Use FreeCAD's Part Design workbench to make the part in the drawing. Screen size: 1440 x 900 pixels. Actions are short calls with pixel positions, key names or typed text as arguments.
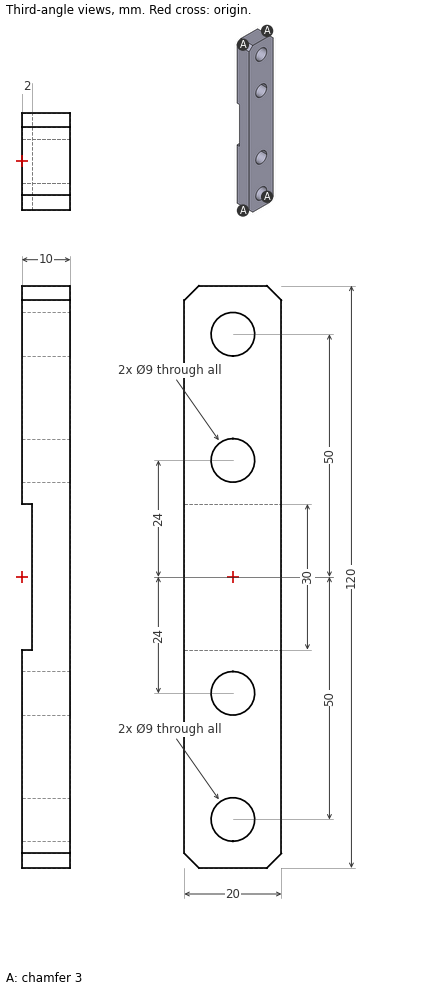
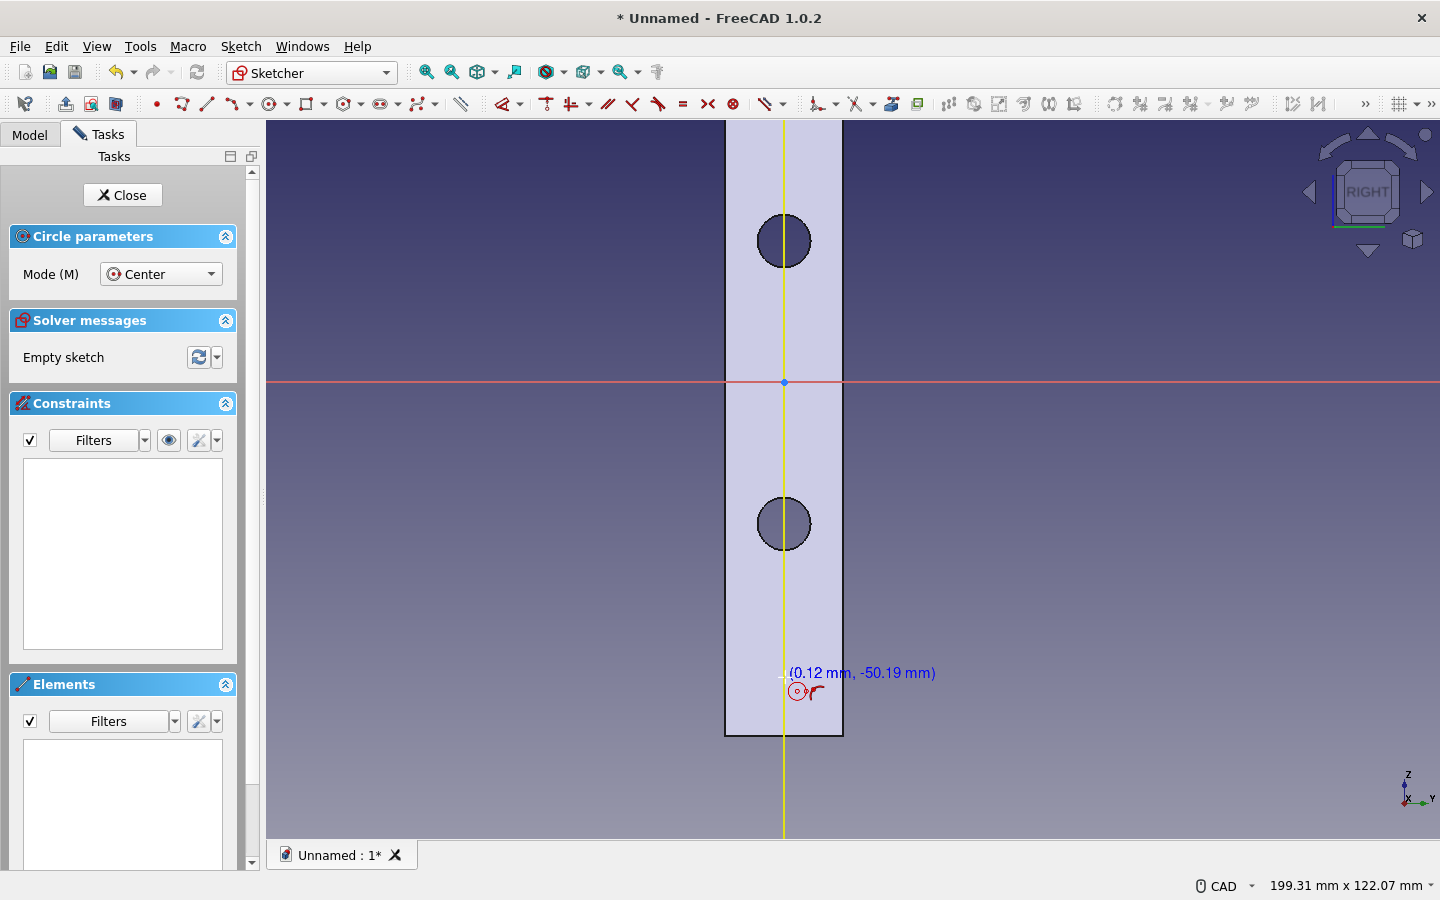
click(784, 677)
move(803, 658)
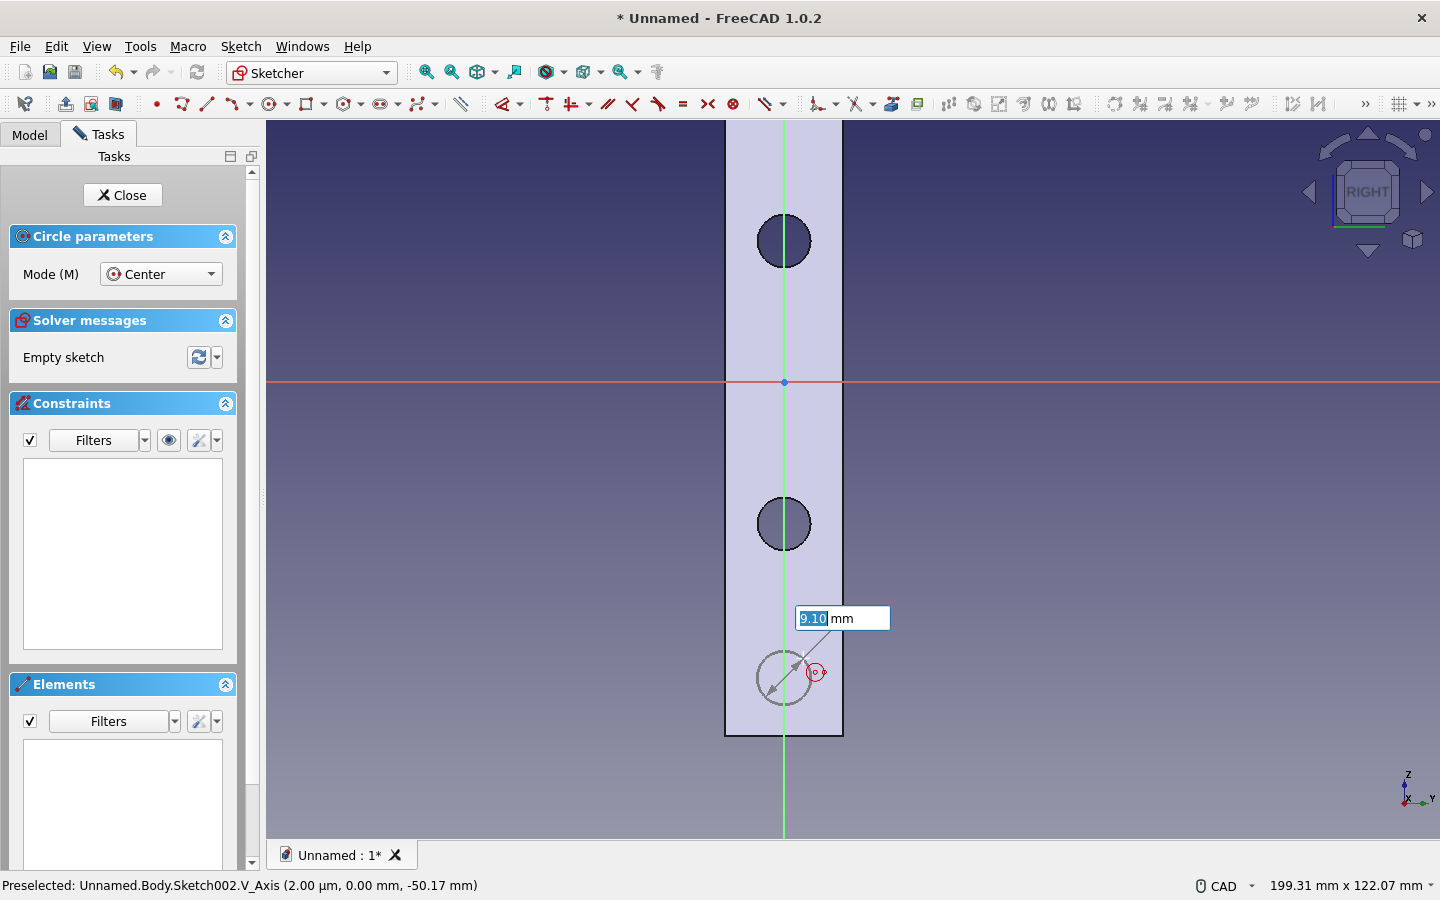
text(9)
key(Return)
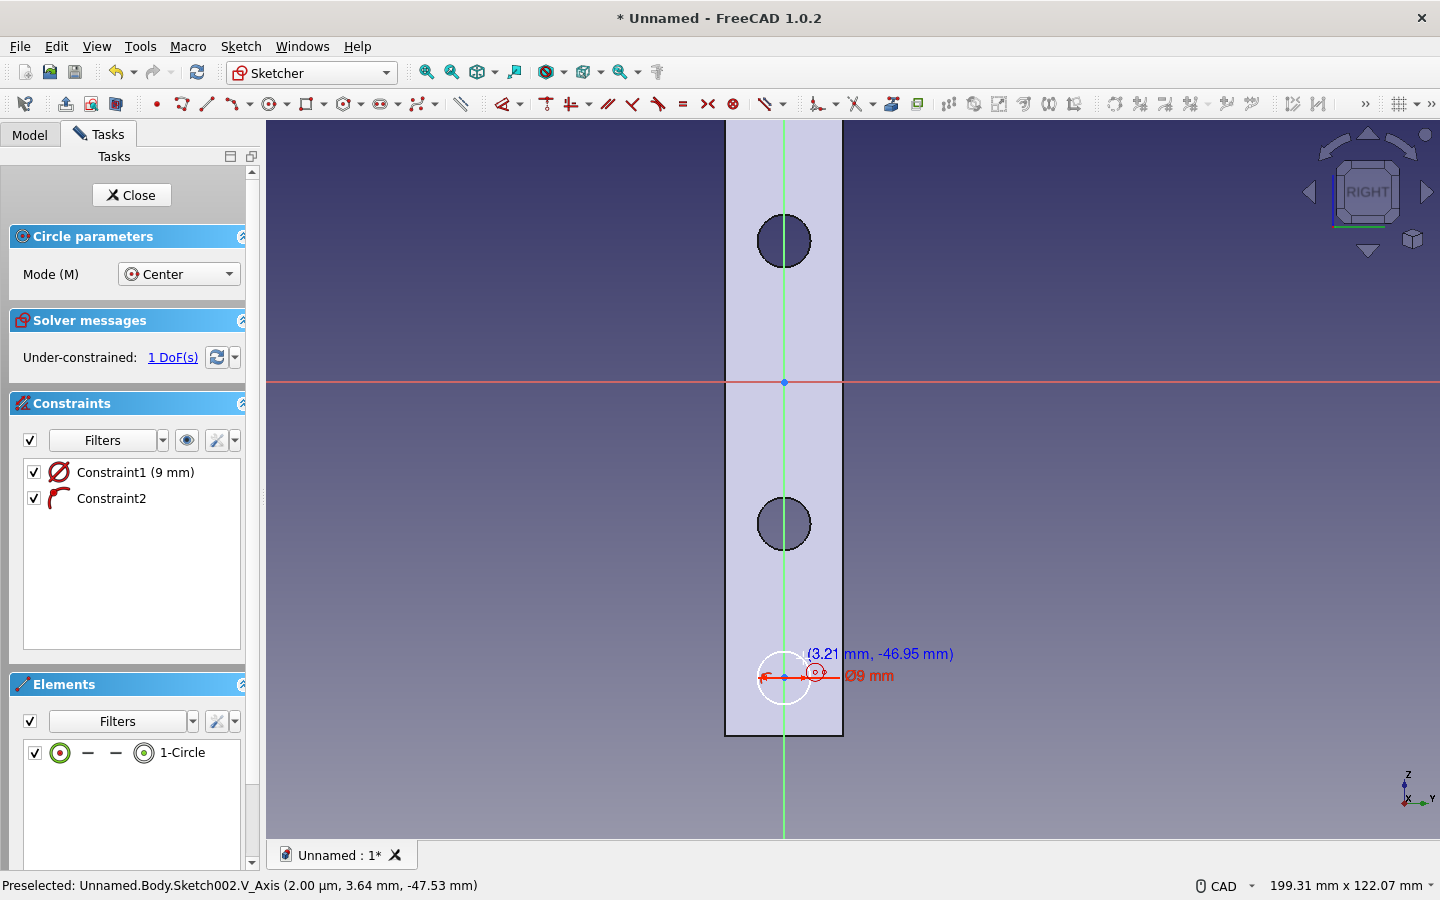
scroll(785, 677, down, 2)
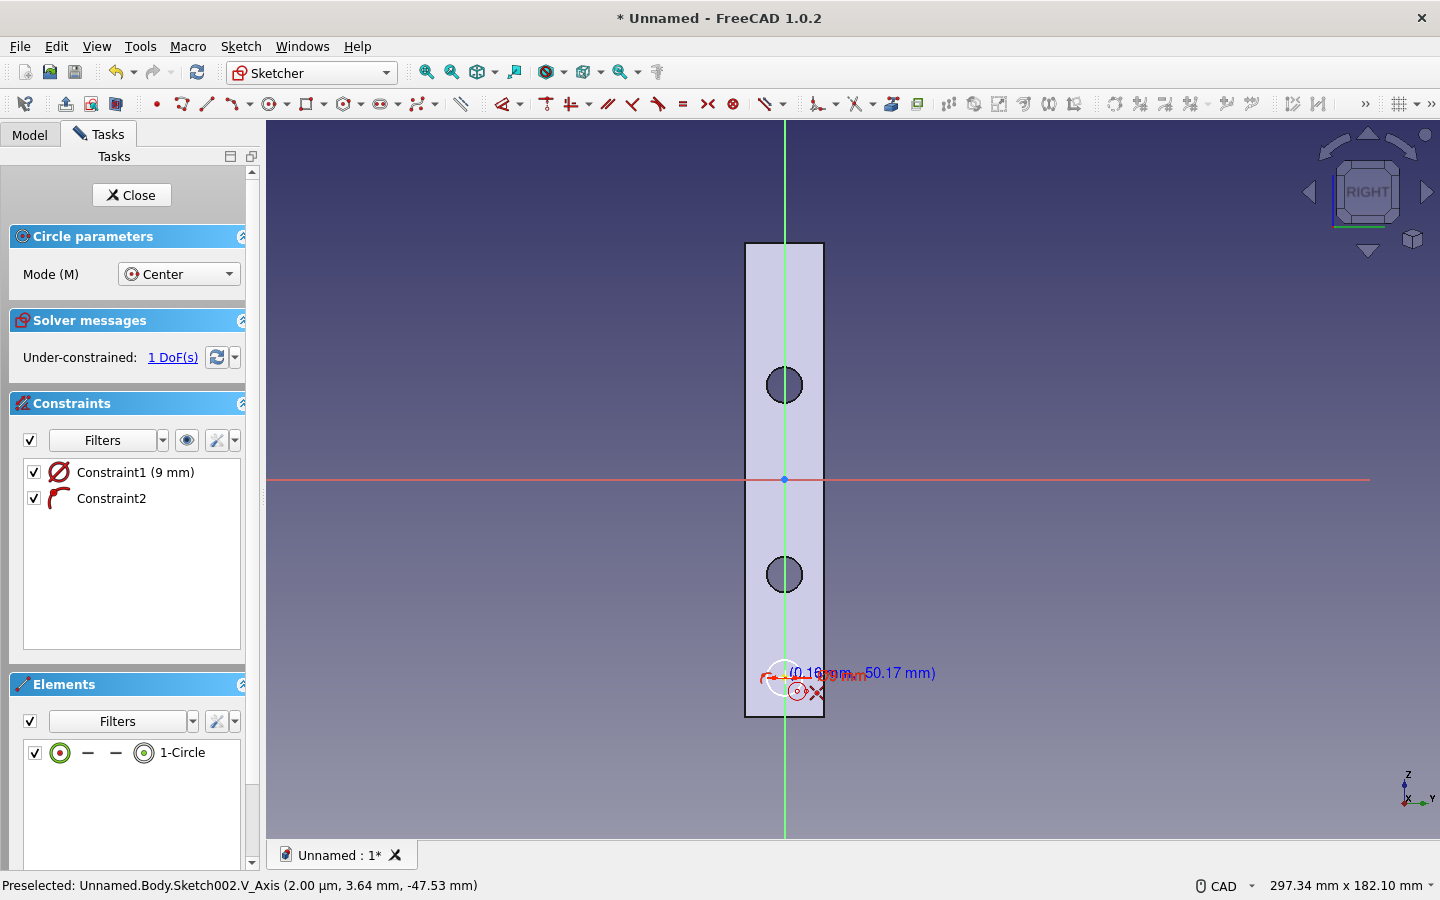
scroll(785, 282, up, 2)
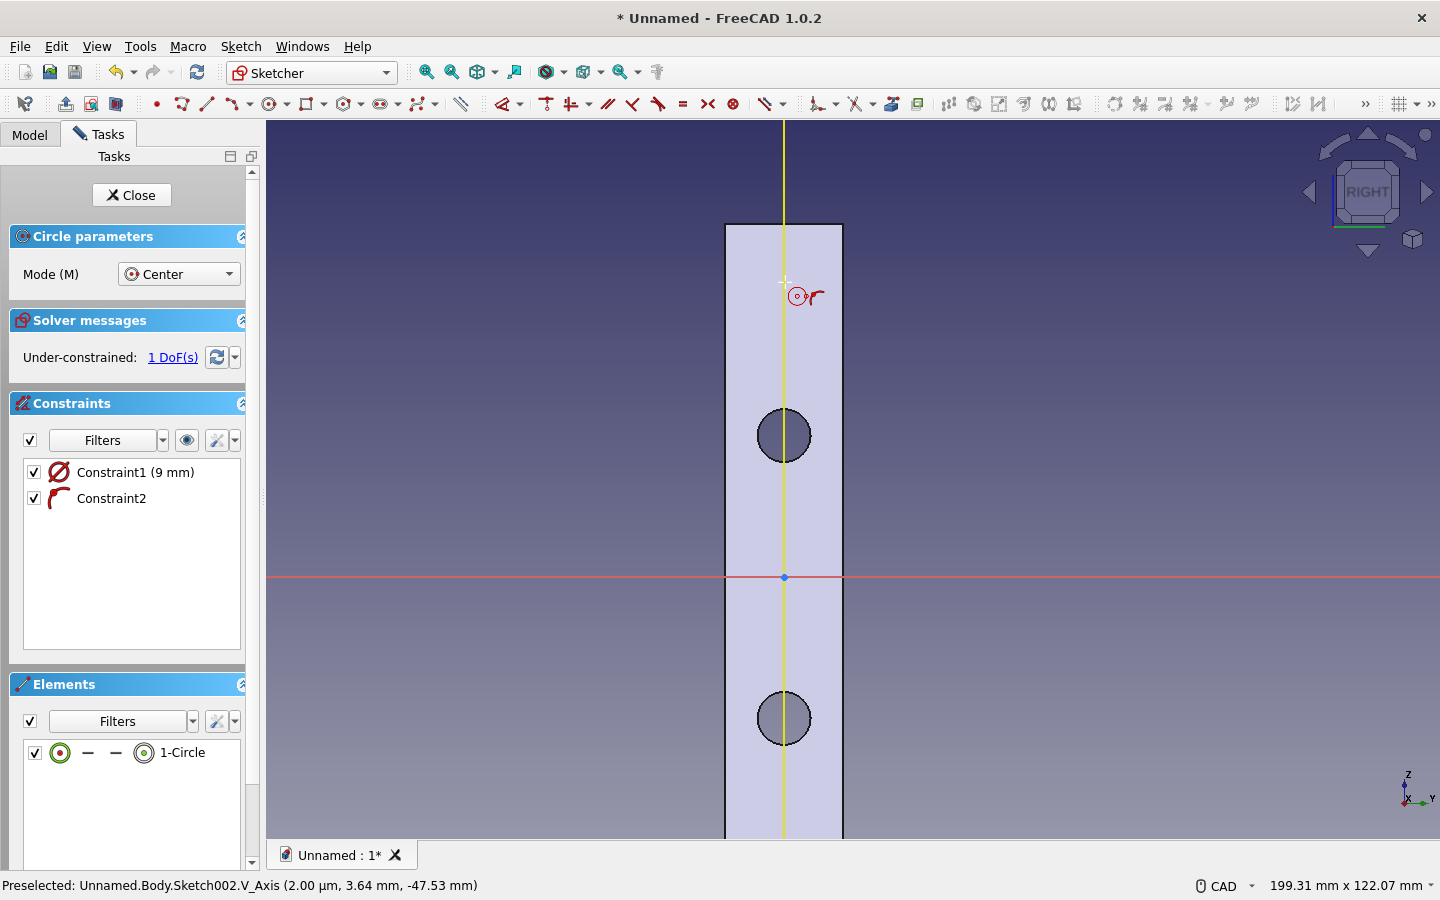
click(784, 283)
move(803, 264)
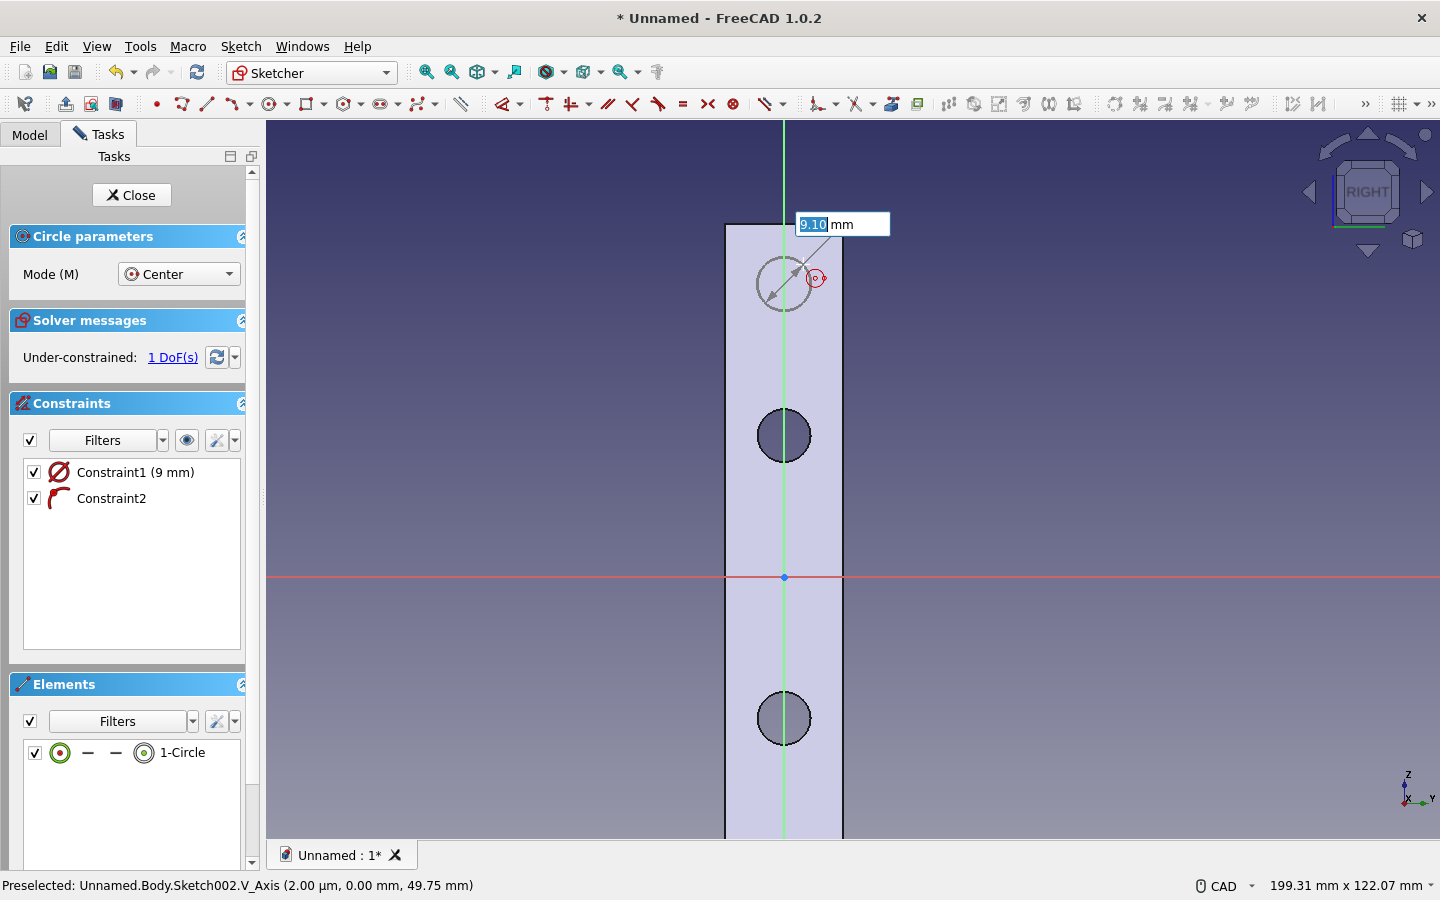
text(9)
key(Return)
key(Escape)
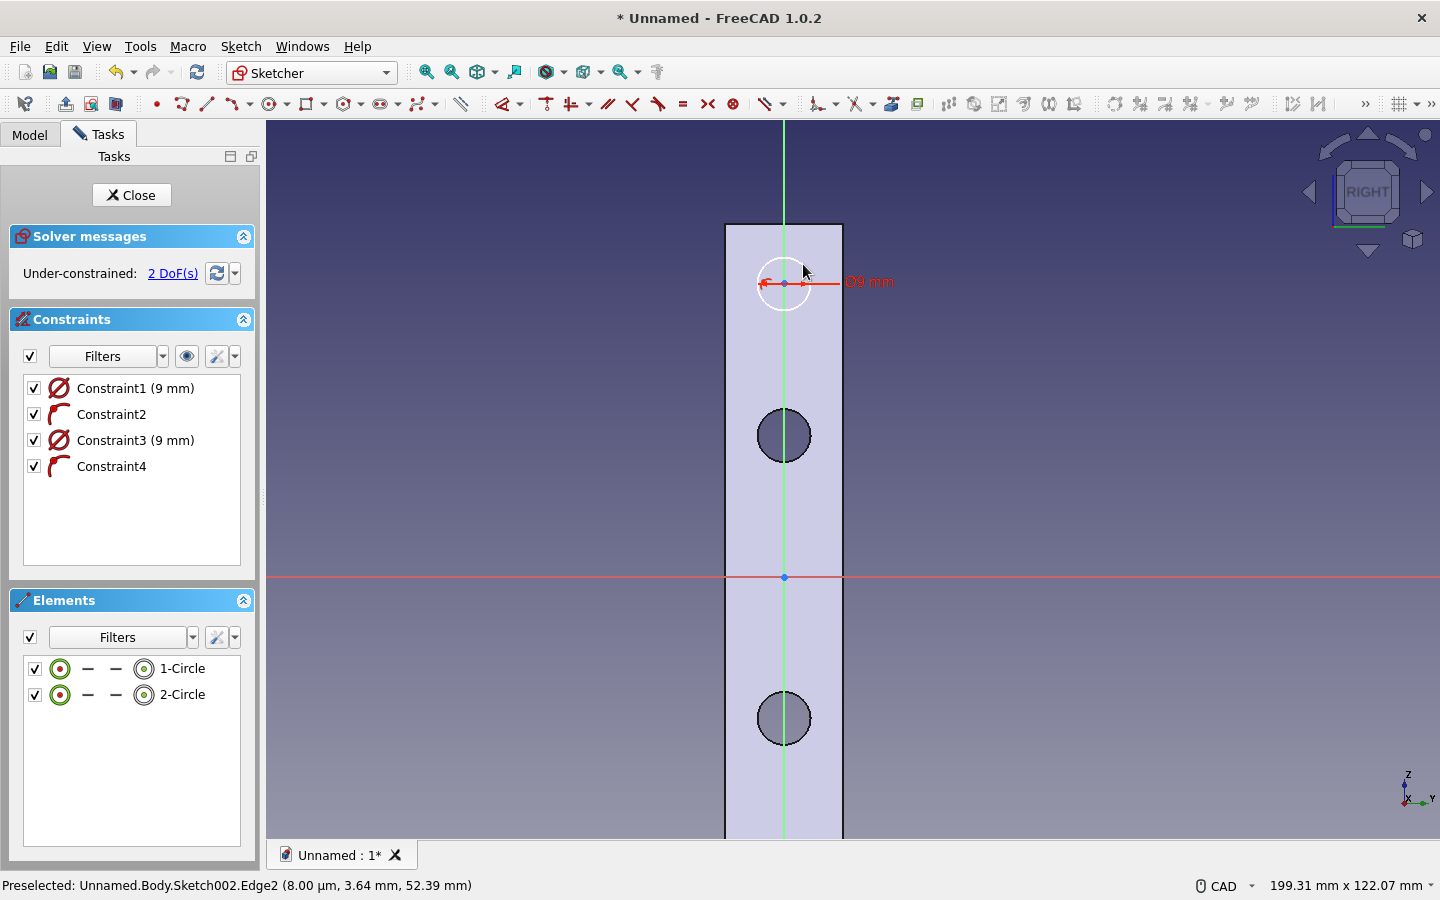
key(d)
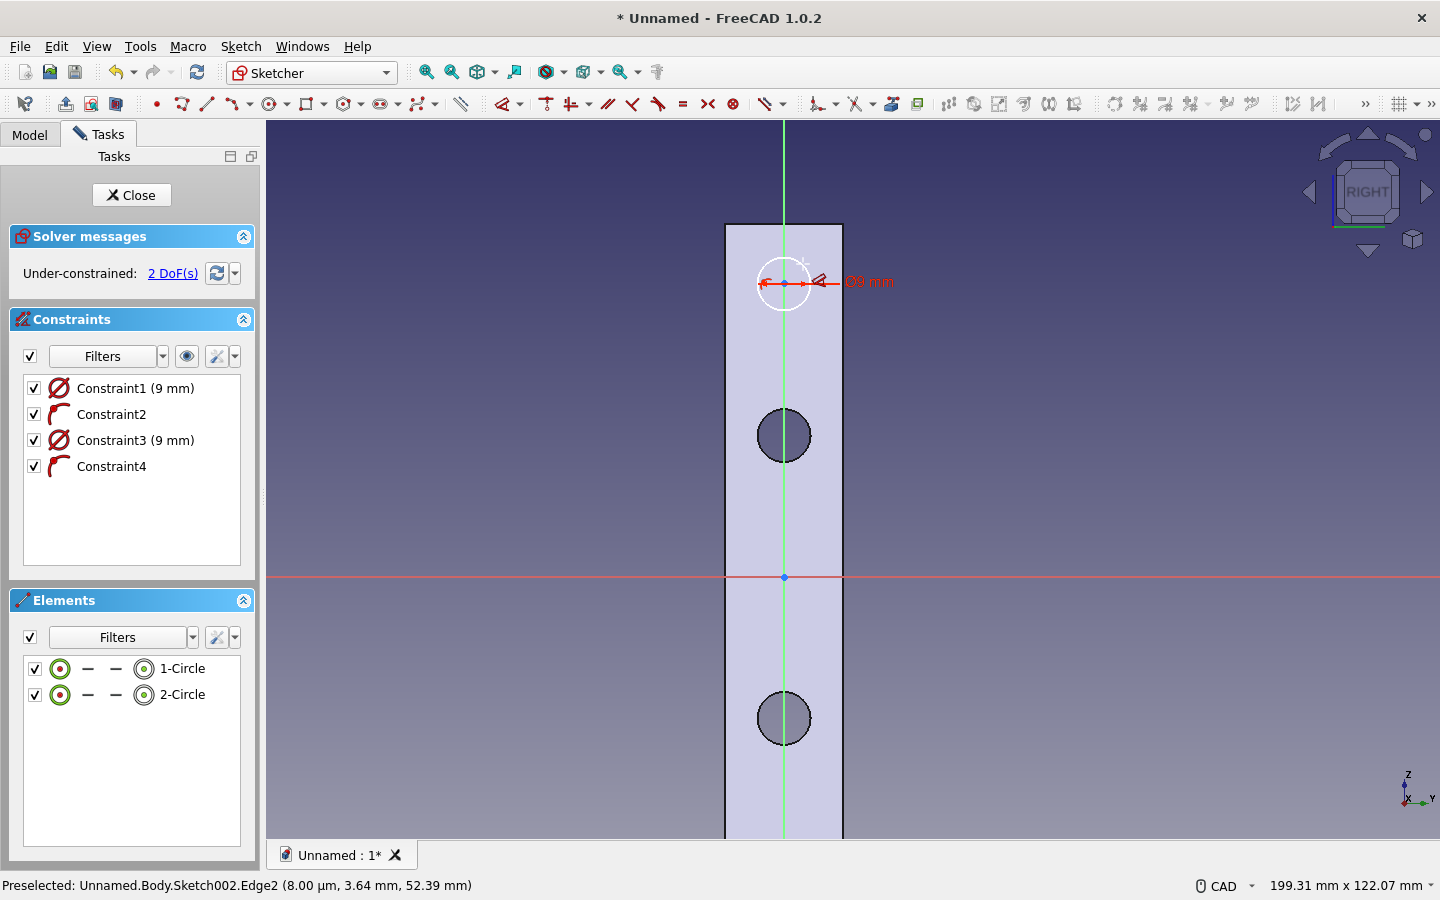
scroll(785, 281, down, 2)